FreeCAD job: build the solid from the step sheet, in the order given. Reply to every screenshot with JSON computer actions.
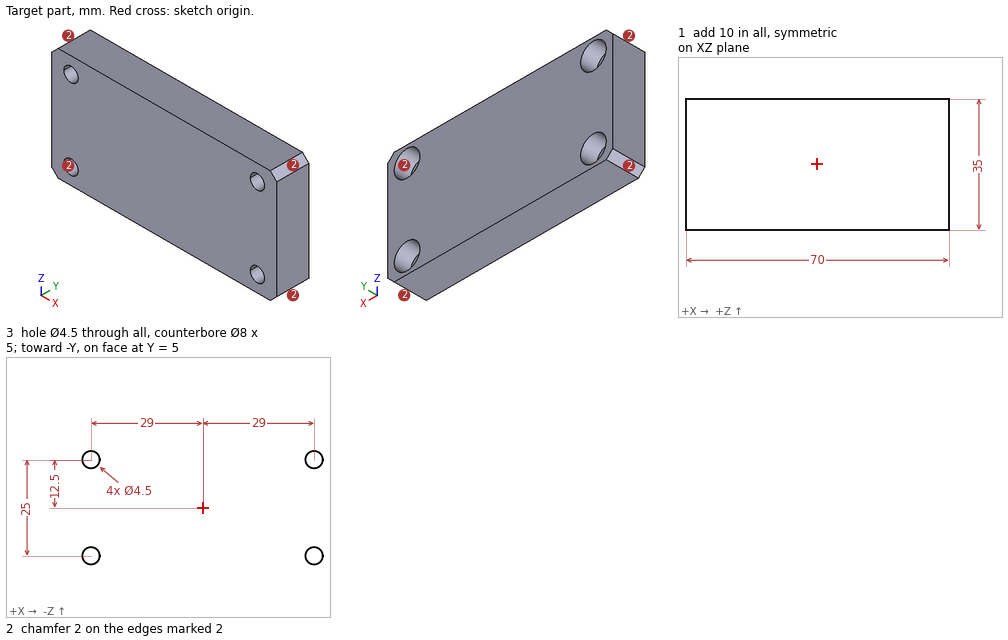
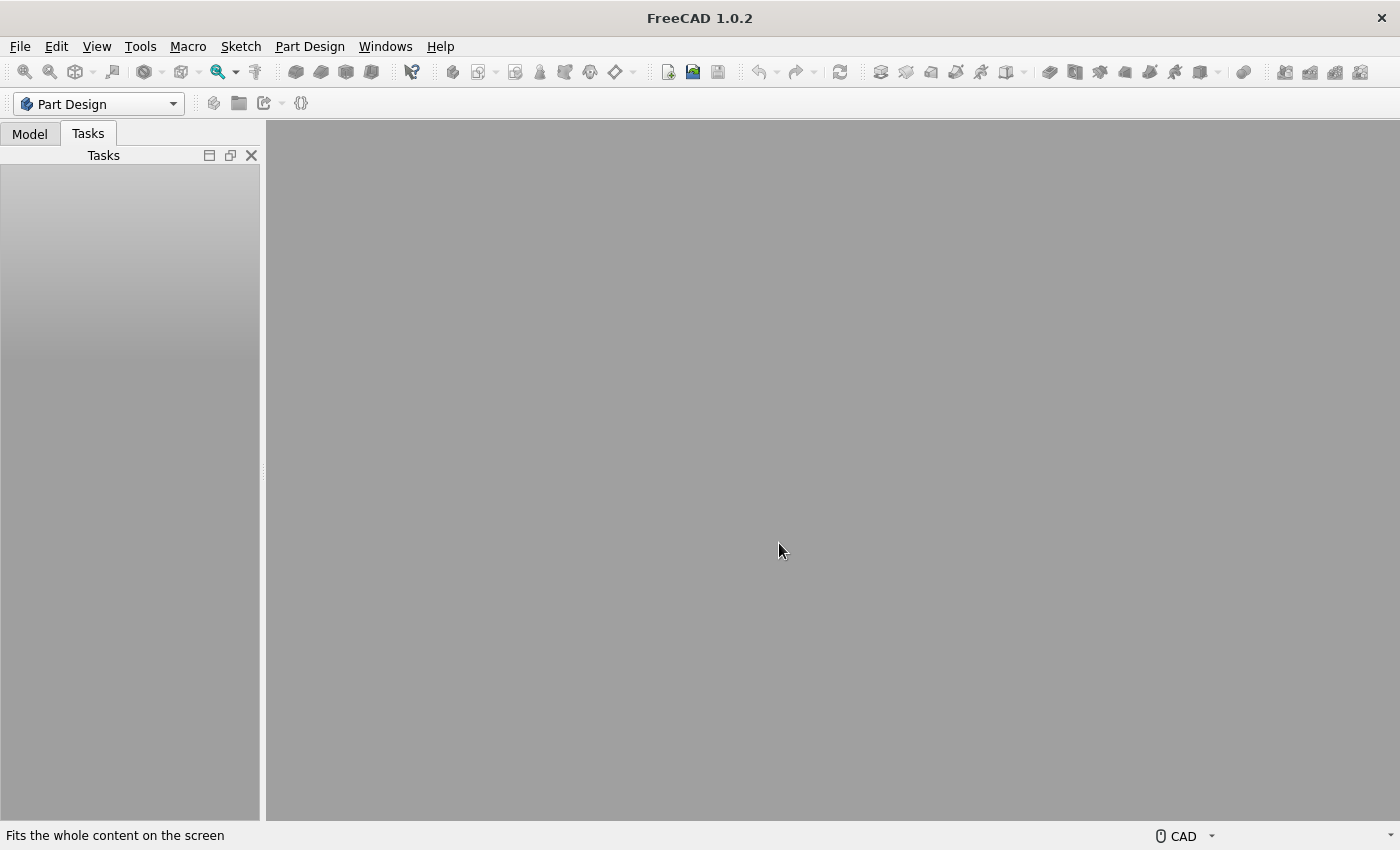
{"action": "left_click", "coordinate": [668, 72]}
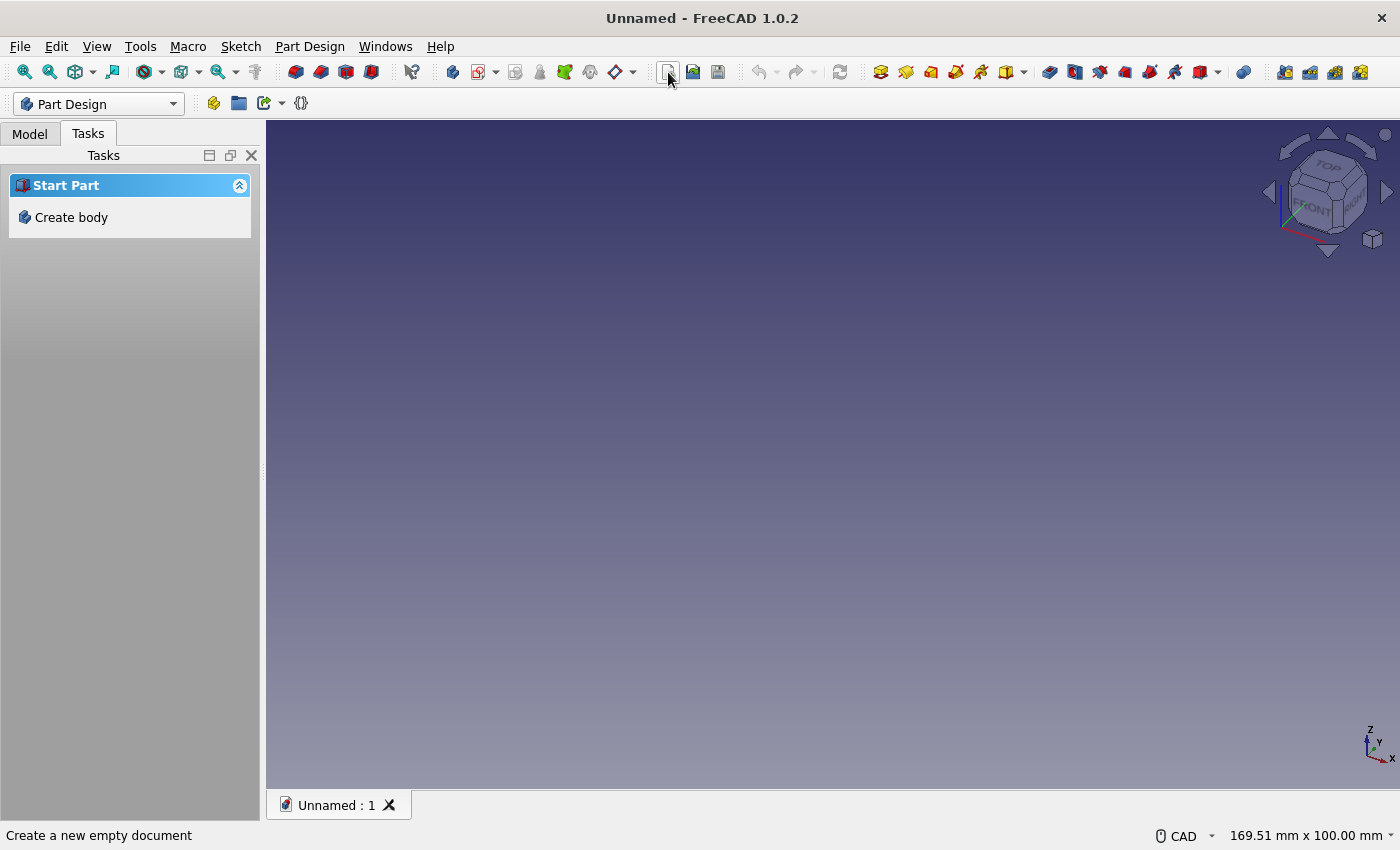
{"action": "left_click", "coordinate": [478, 72]}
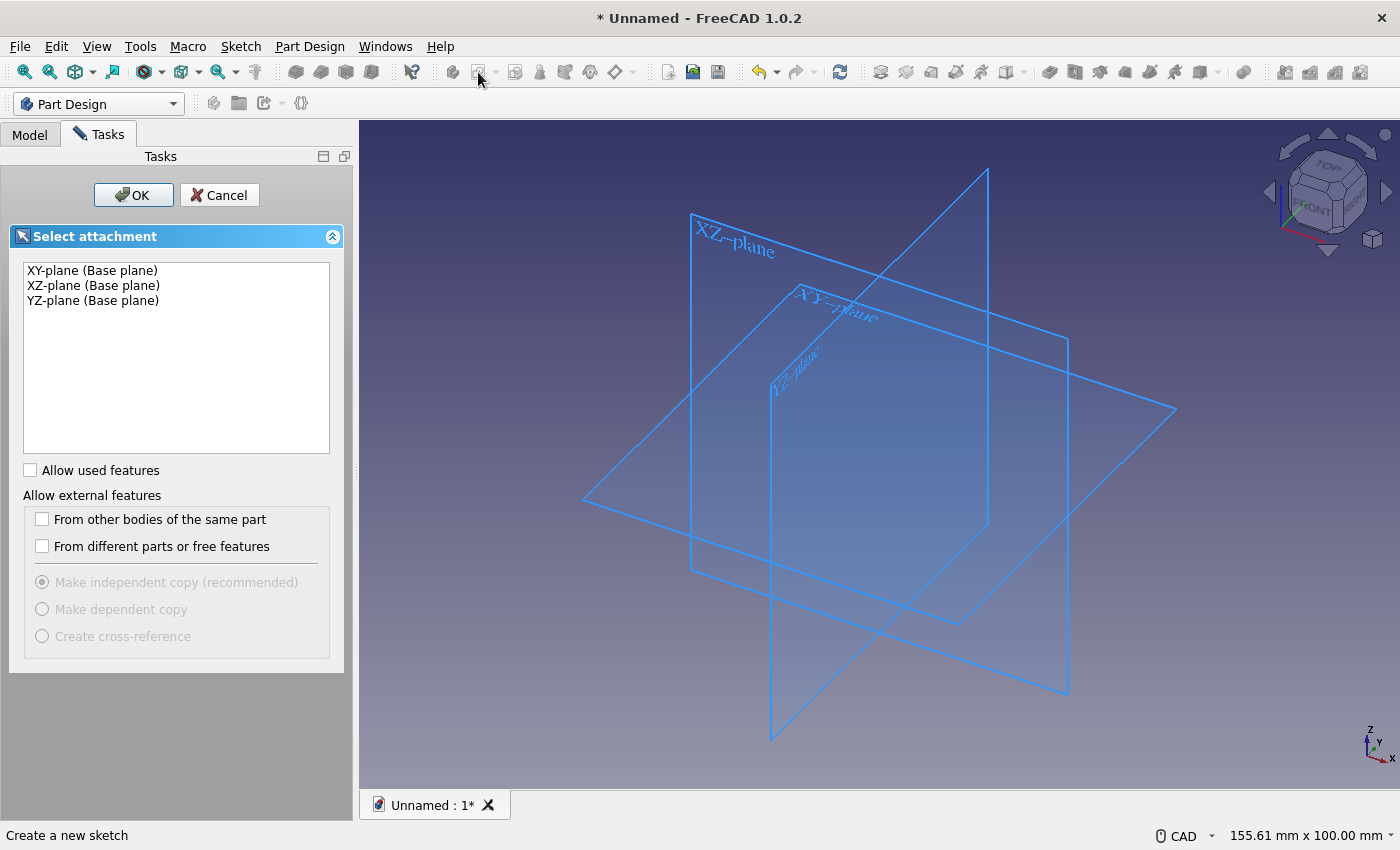
{"action": "left_click", "coordinate": [84, 286]}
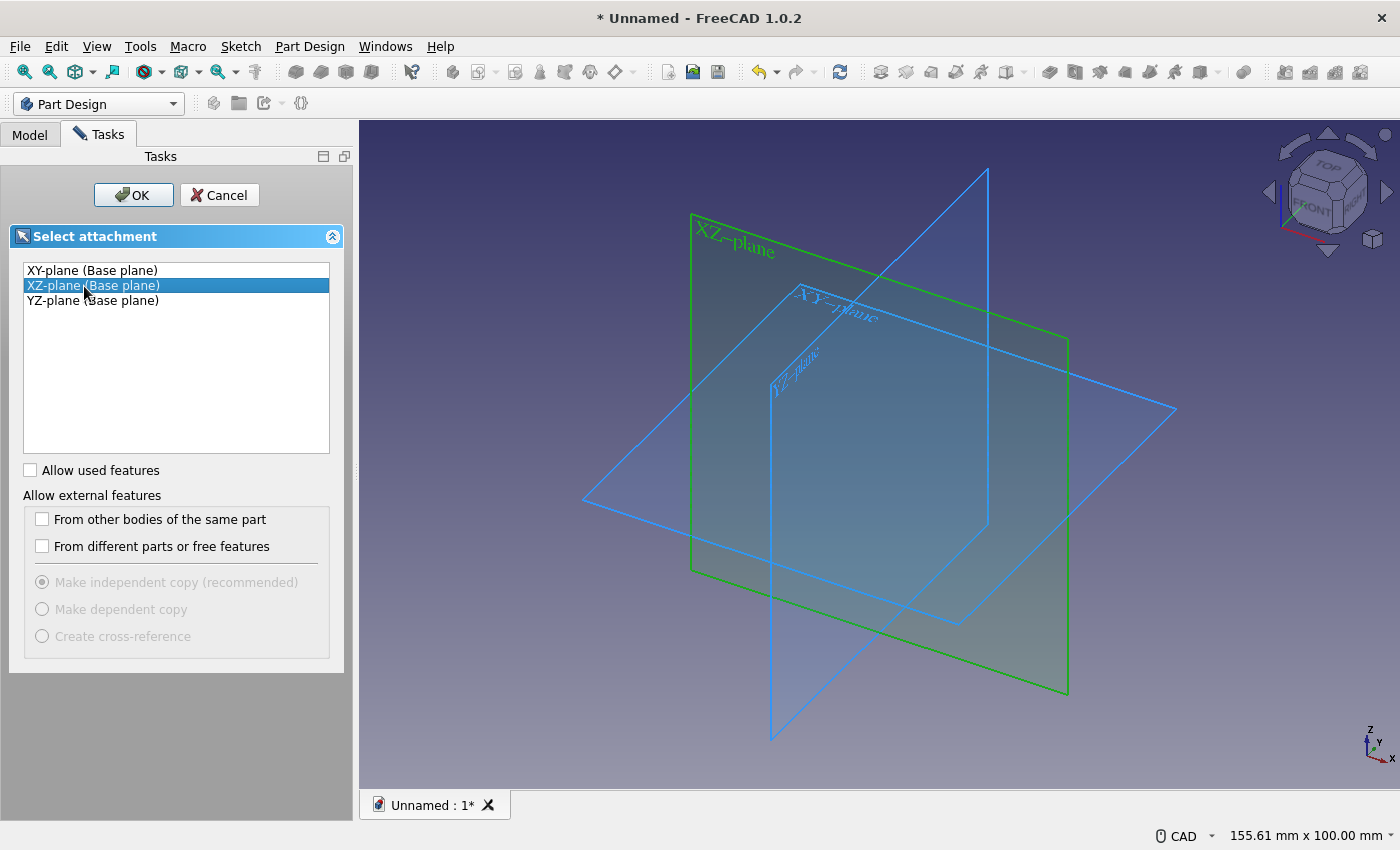
{"action": "left_click", "coordinate": [134, 195]}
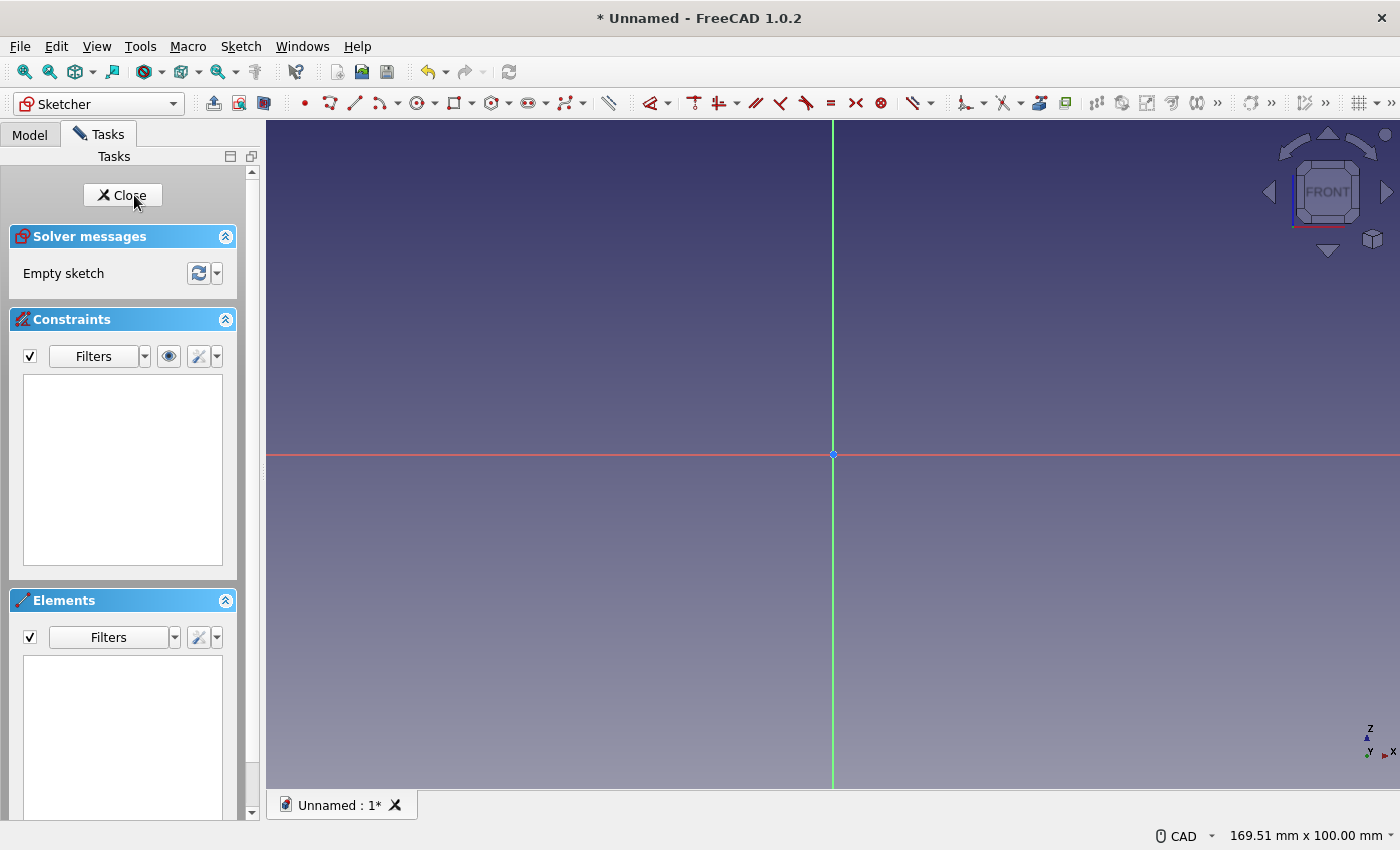
{"action": "scroll", "coordinate": [972, 455], "scroll_direction": "up", "scroll_amount": 2}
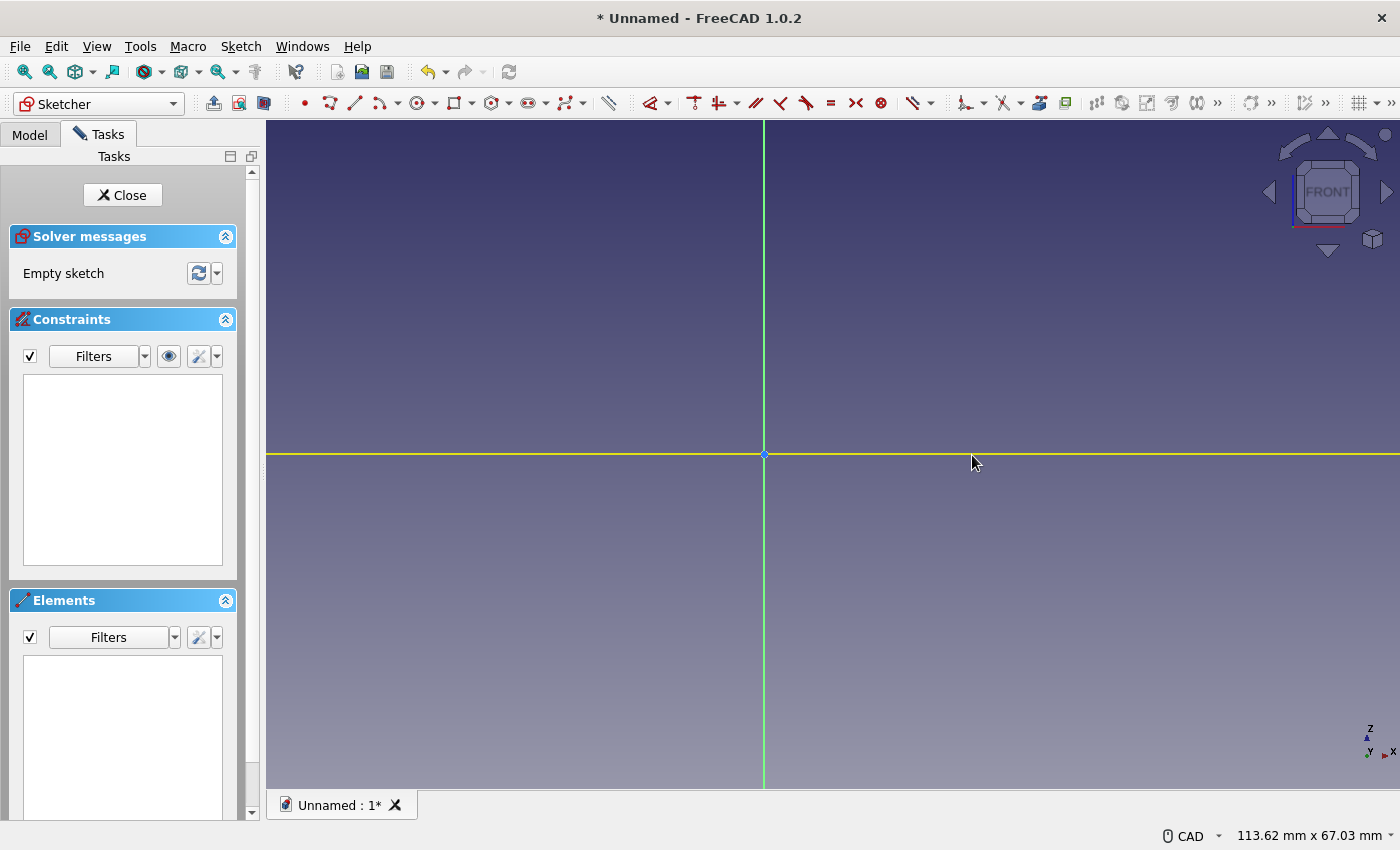
{"action": "key", "text": "g v"}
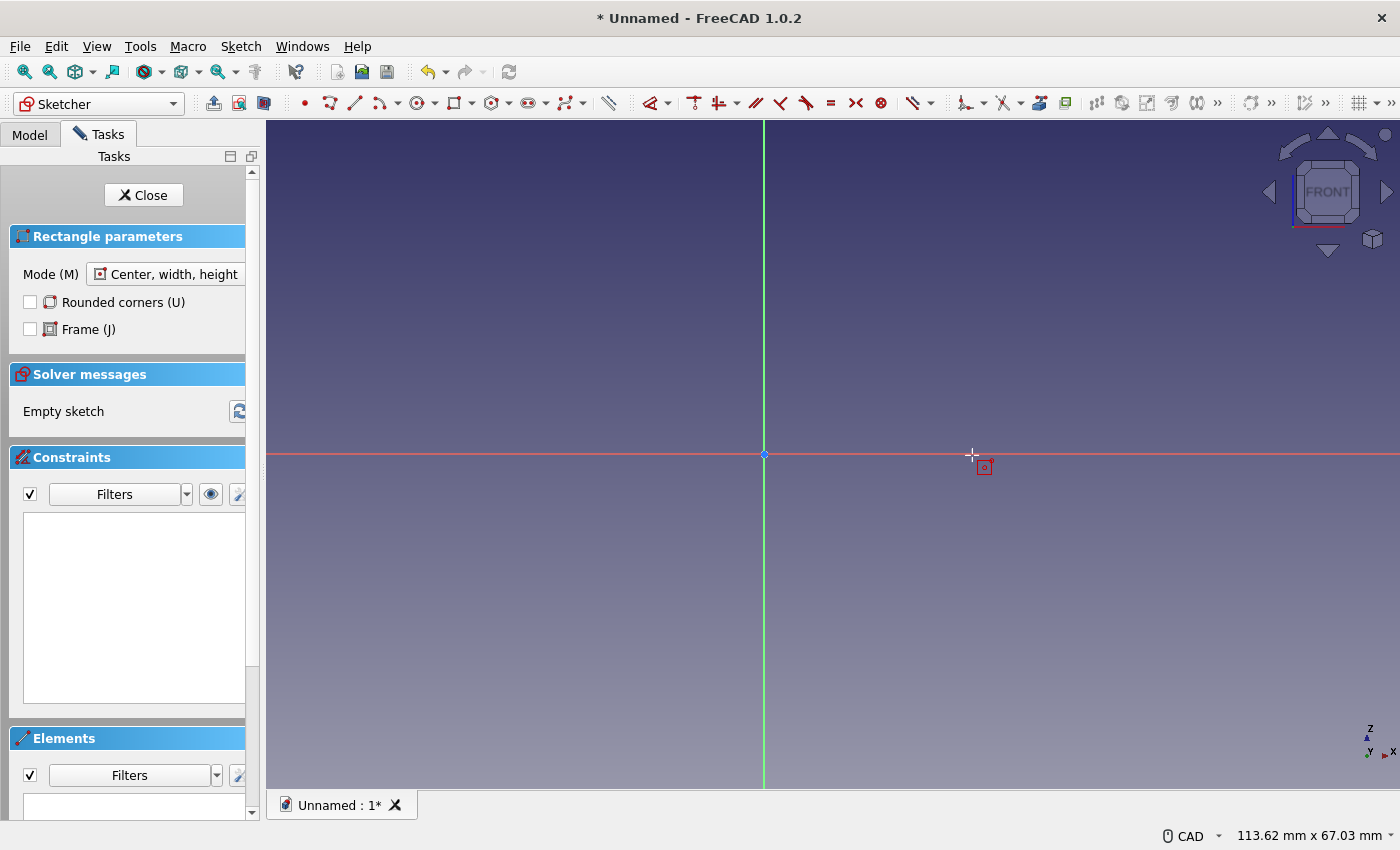
{"action": "left_click", "coordinate": [764, 454]}
{"action": "left_click", "coordinate": [1114, 279]}
{"action": "key", "text": "Escape"}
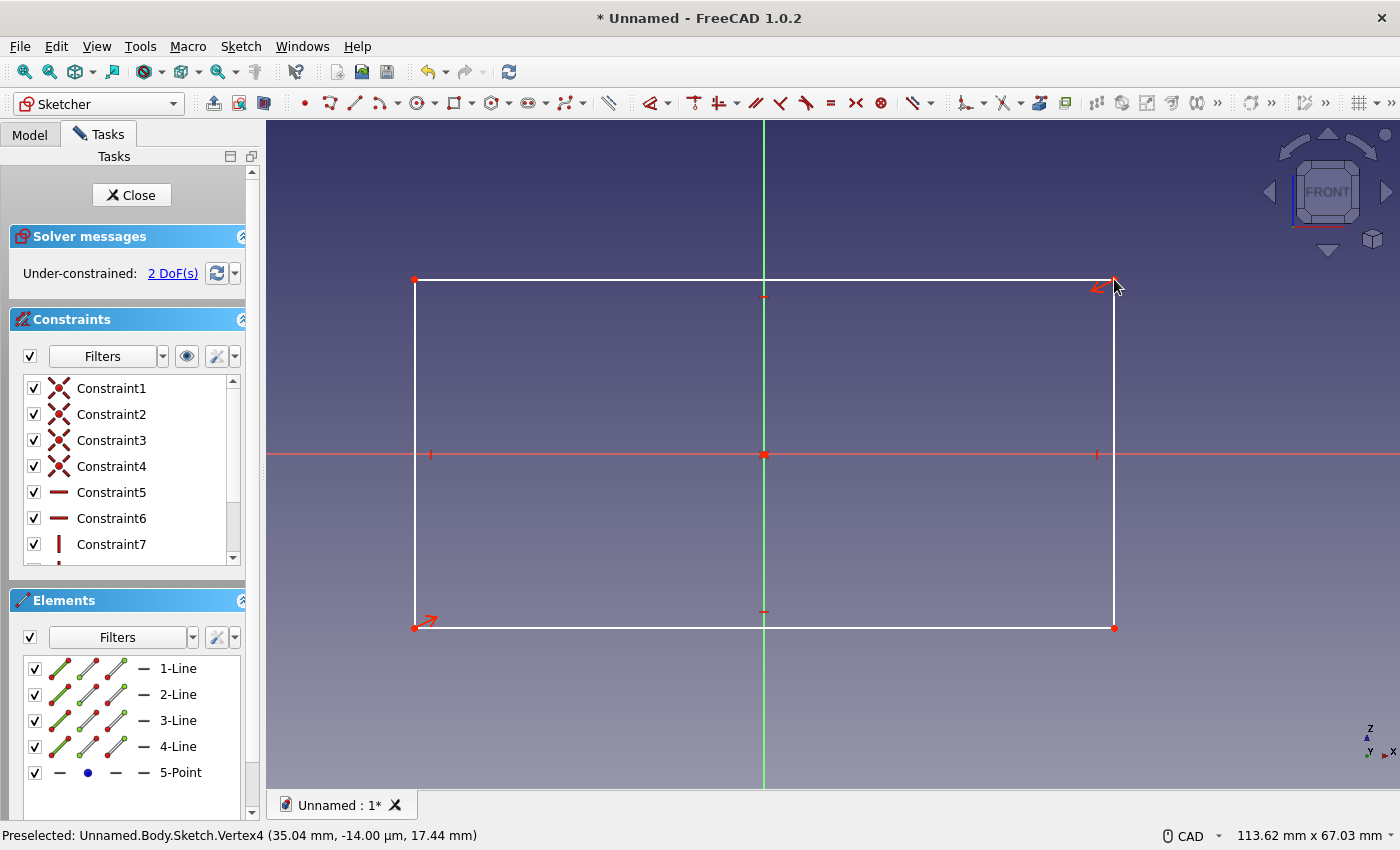
{"action": "left_click", "coordinate": [624, 628]}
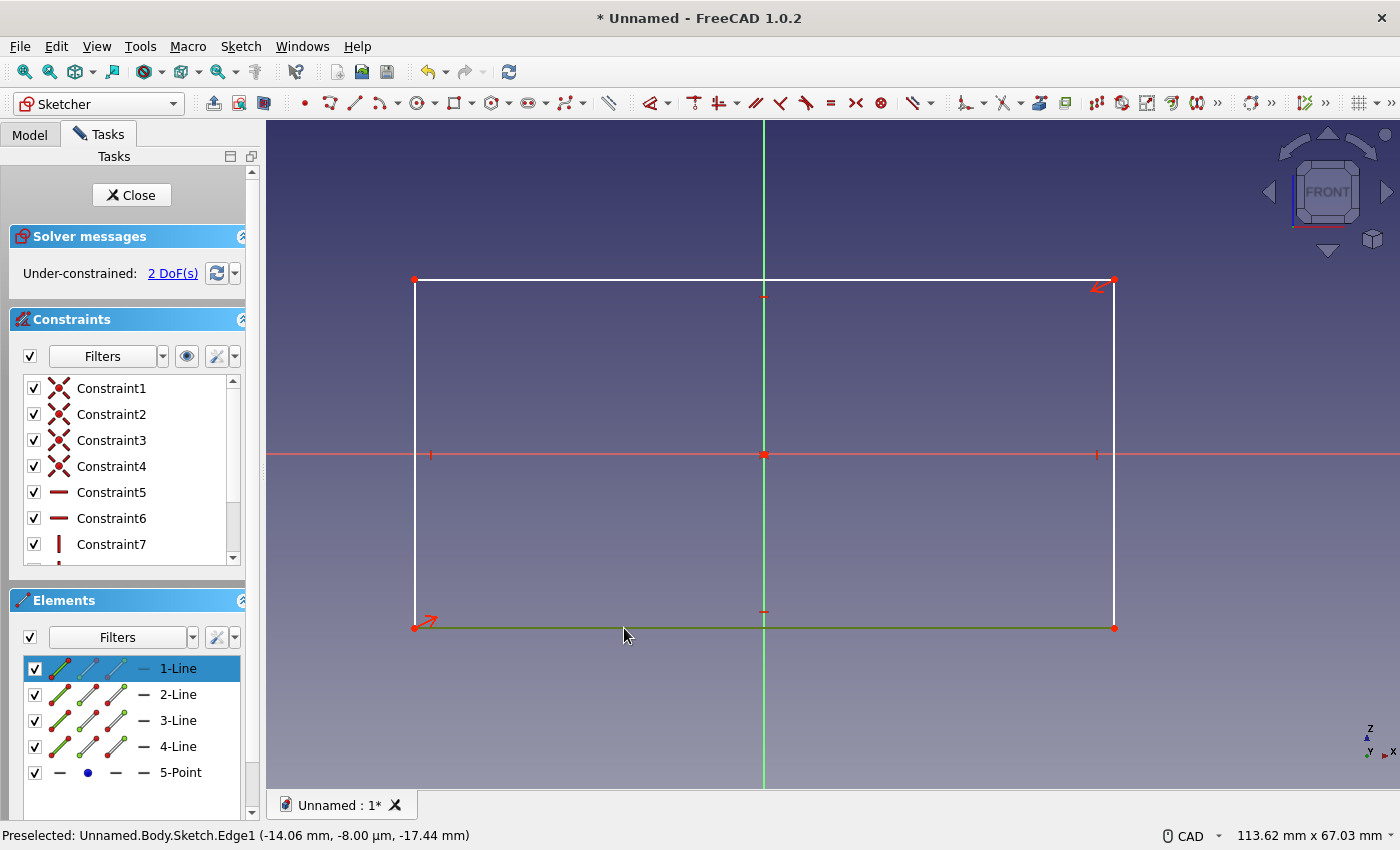
{"action": "left_click", "coordinate": [668, 104]}